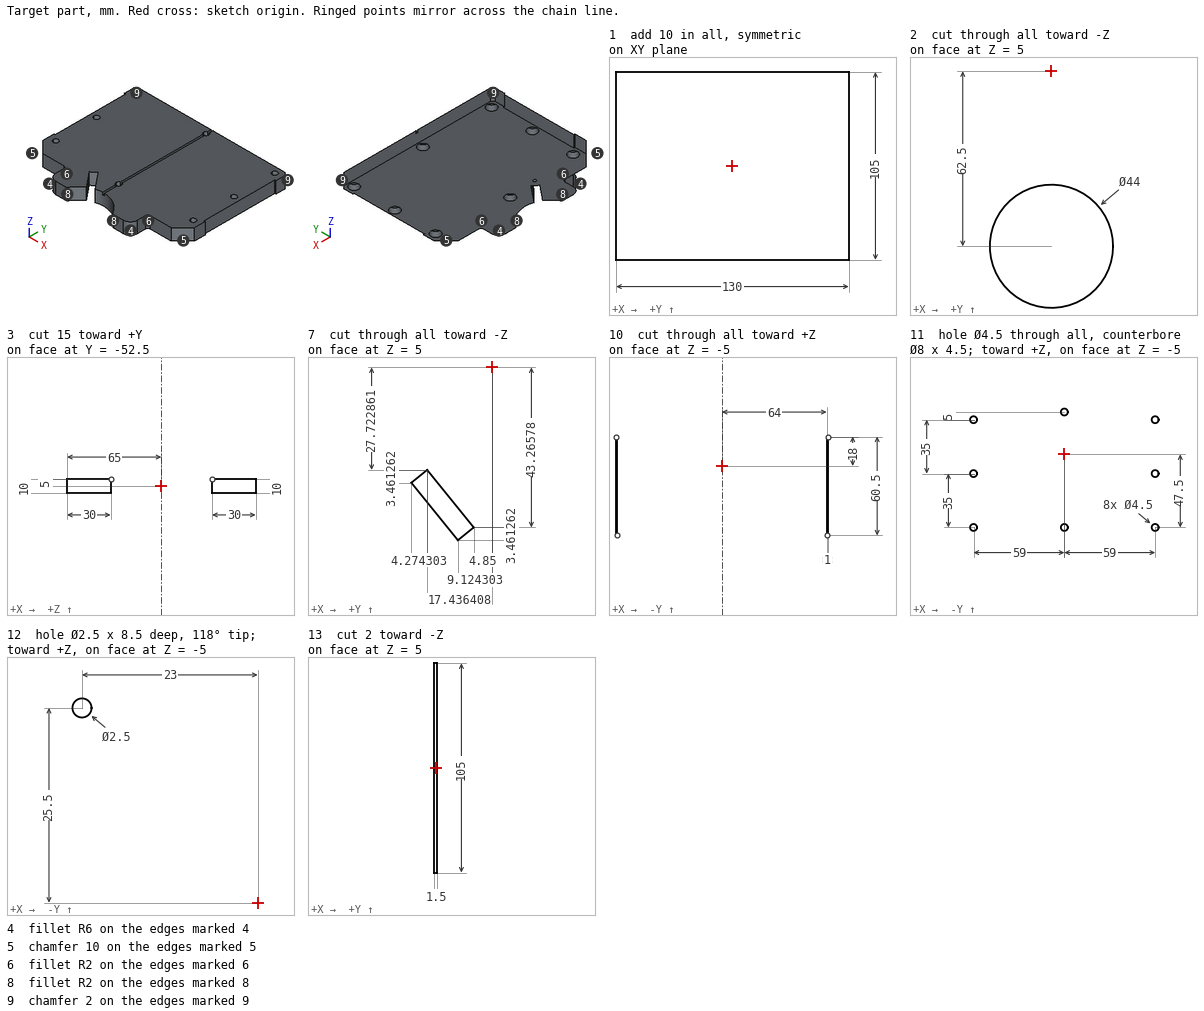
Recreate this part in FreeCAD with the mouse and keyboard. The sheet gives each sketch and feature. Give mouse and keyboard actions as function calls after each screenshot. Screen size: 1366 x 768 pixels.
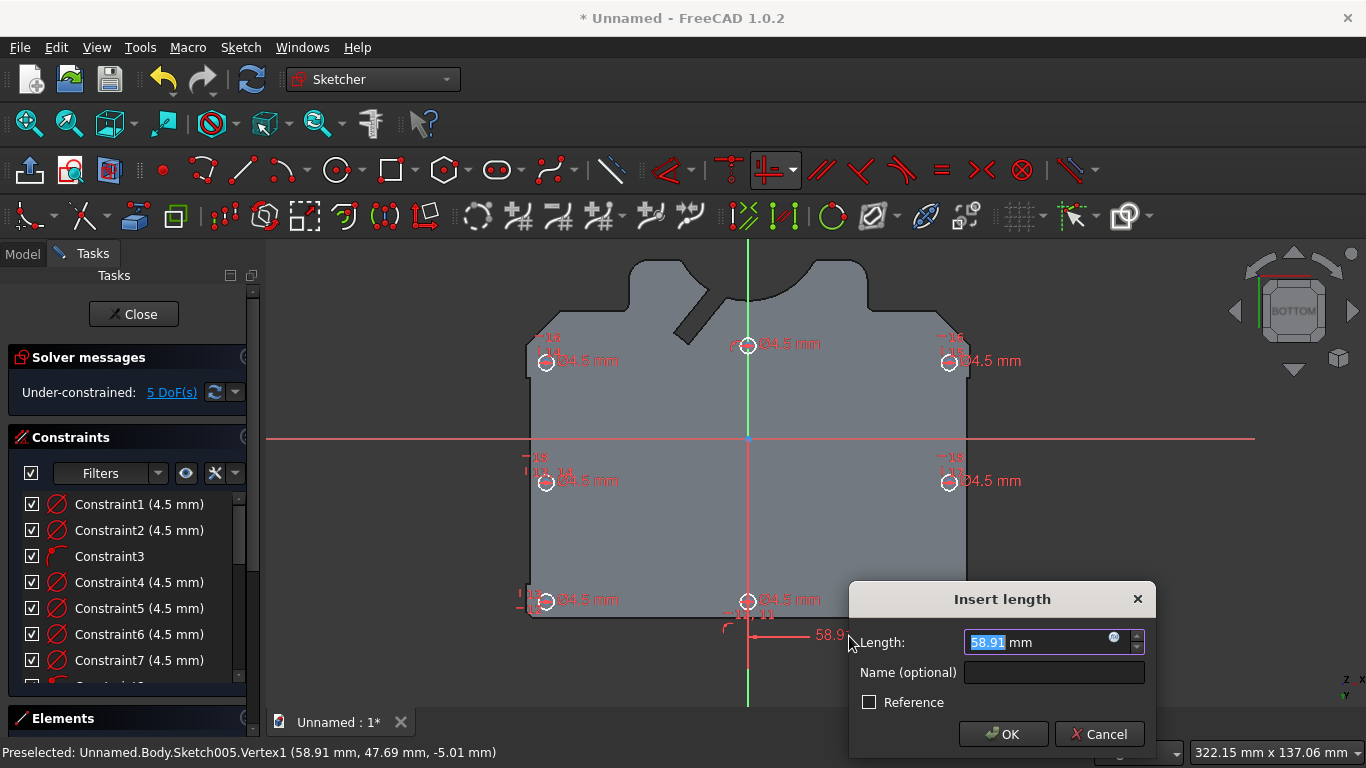
text(59)
key(Return)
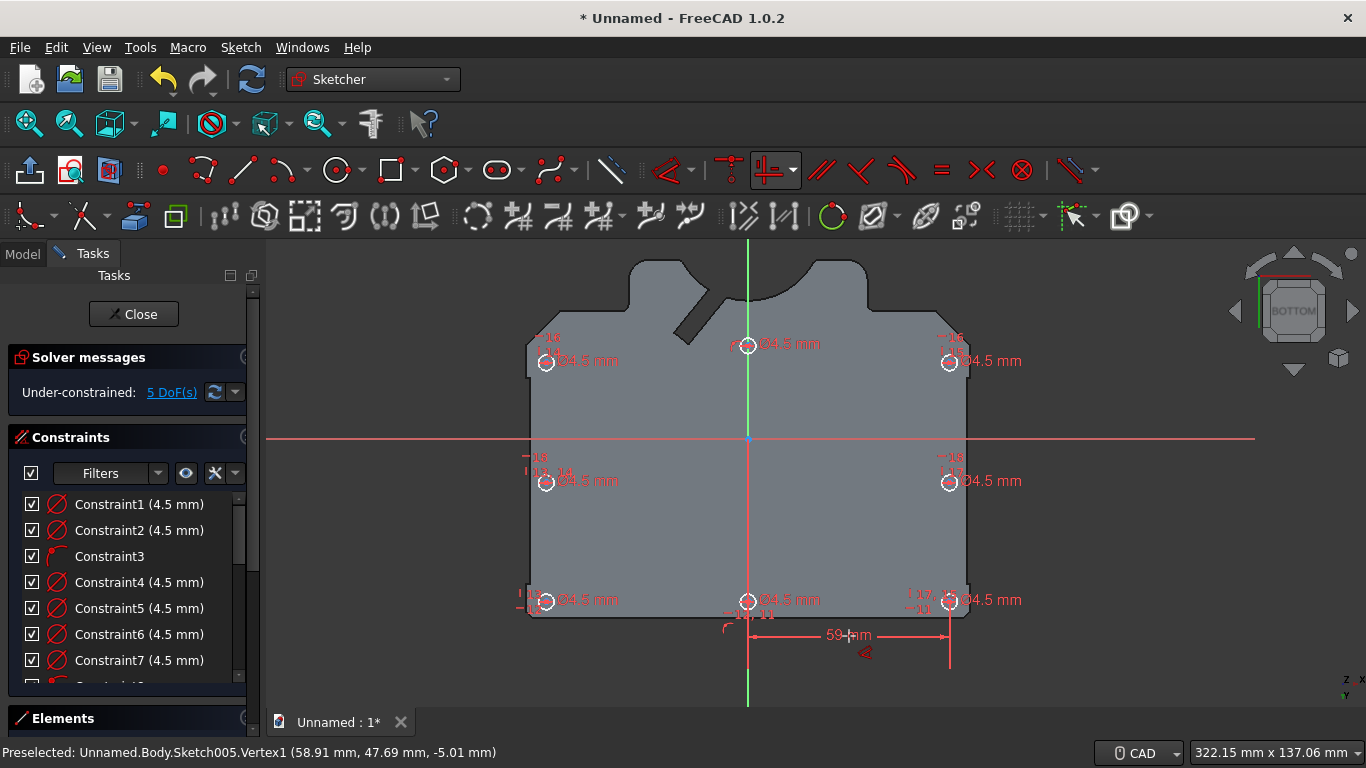
click(546, 602)
click(647, 636)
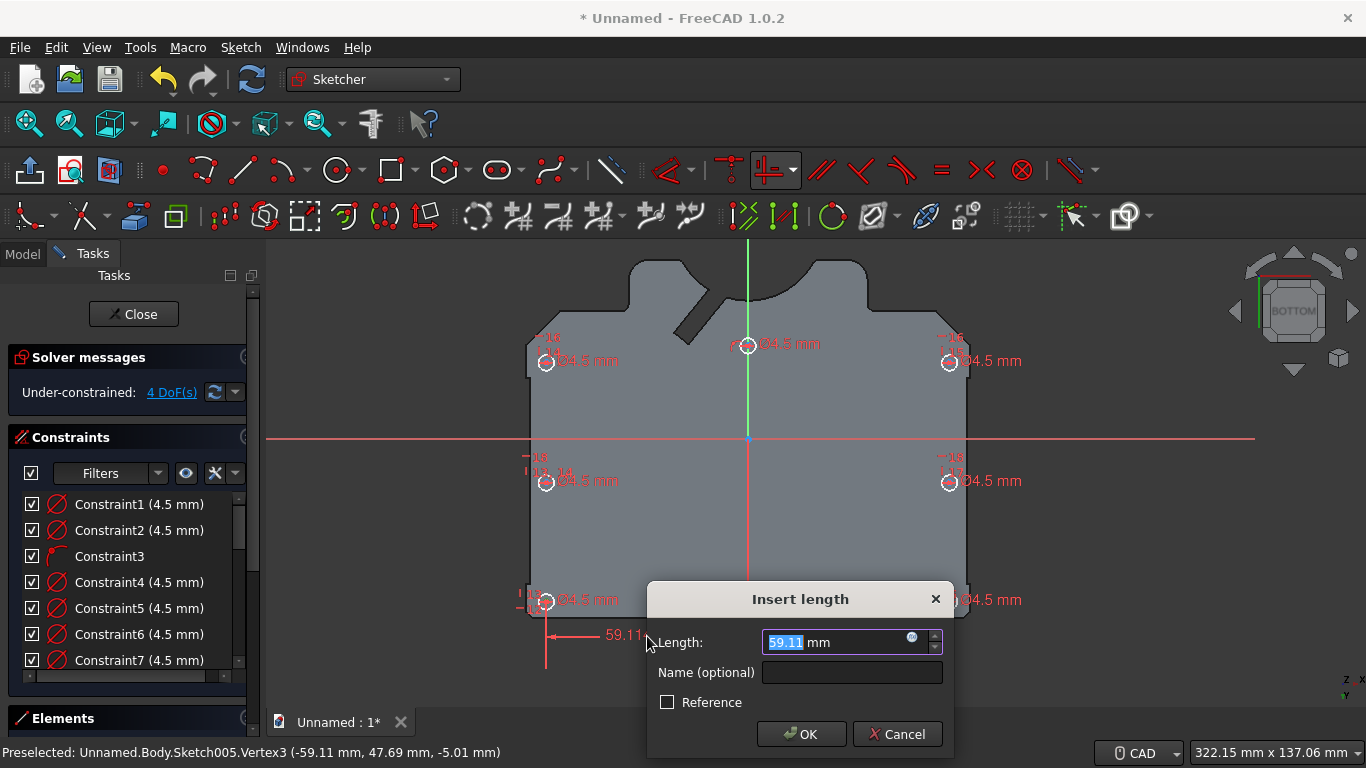
text(59)
key(Return)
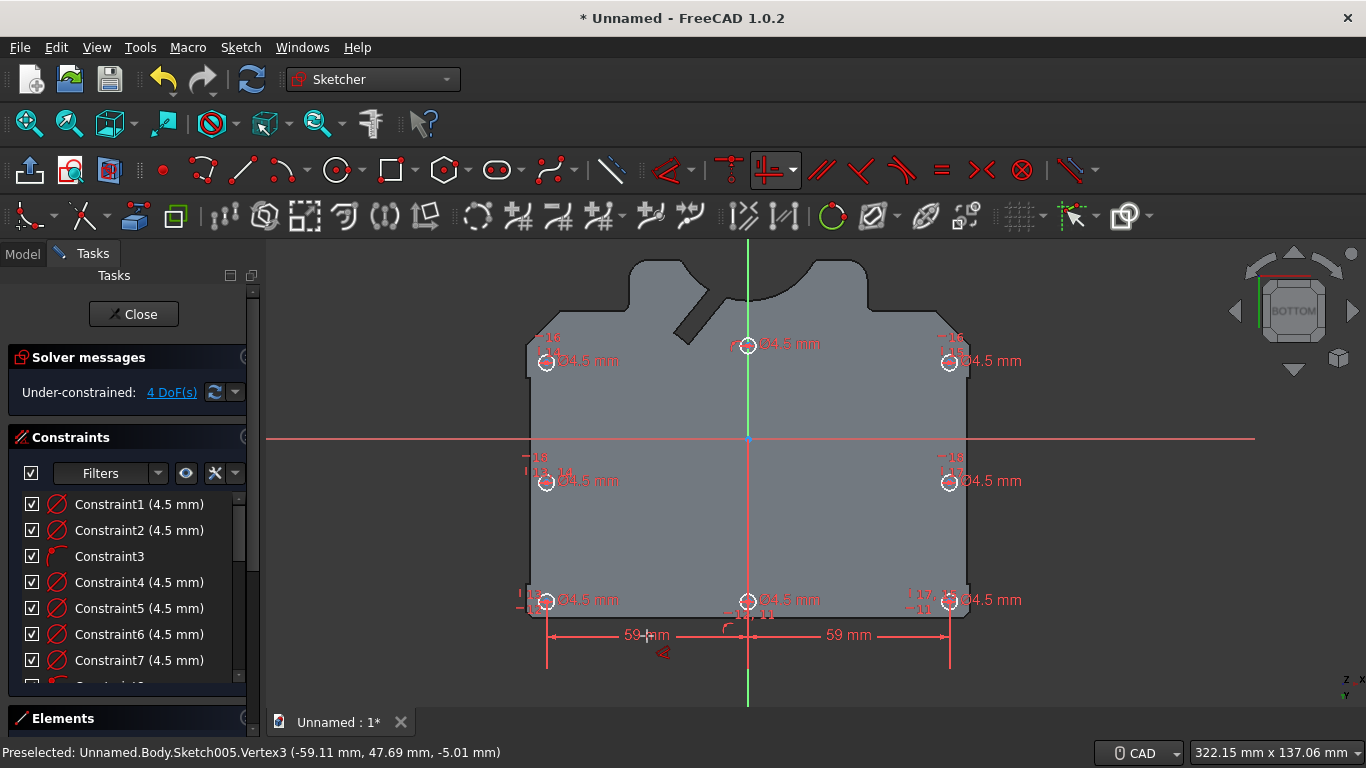
scroll(547, 363, up, 5)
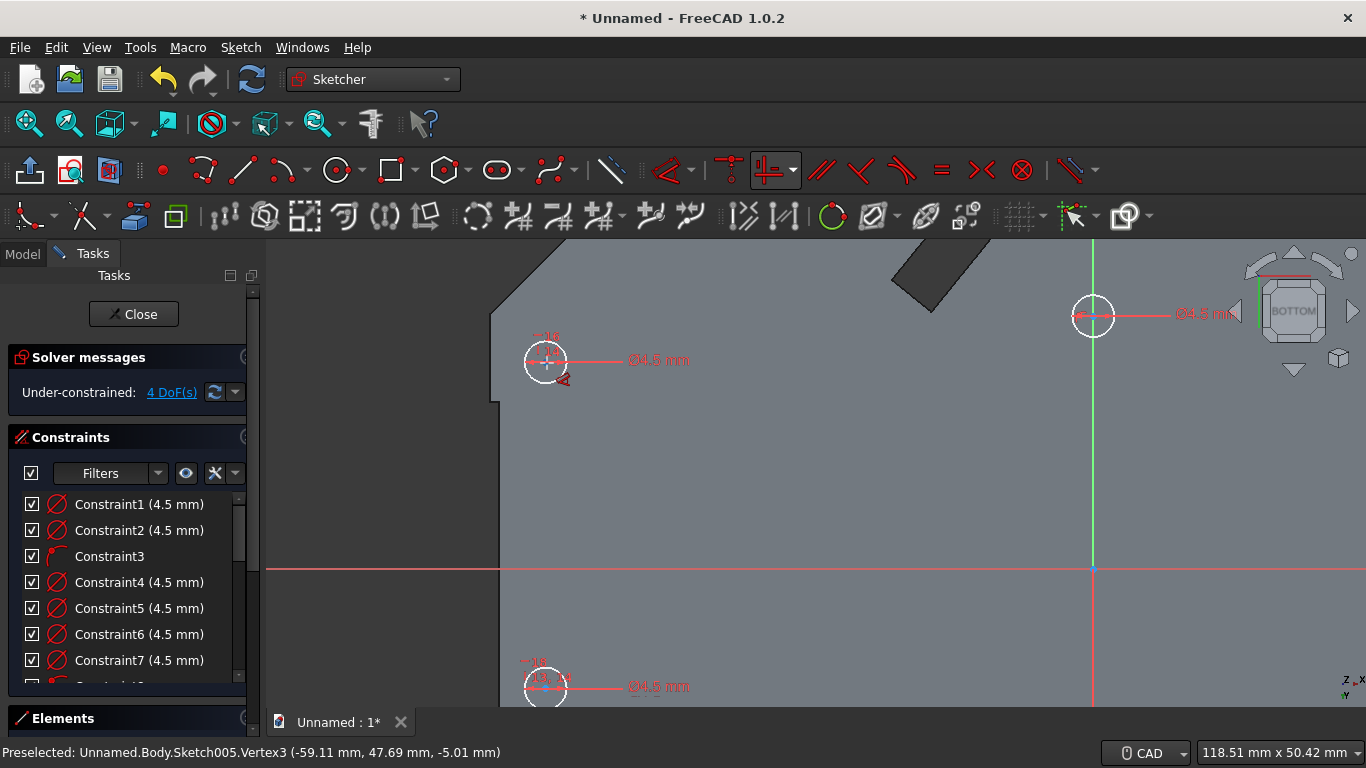
click(546, 362)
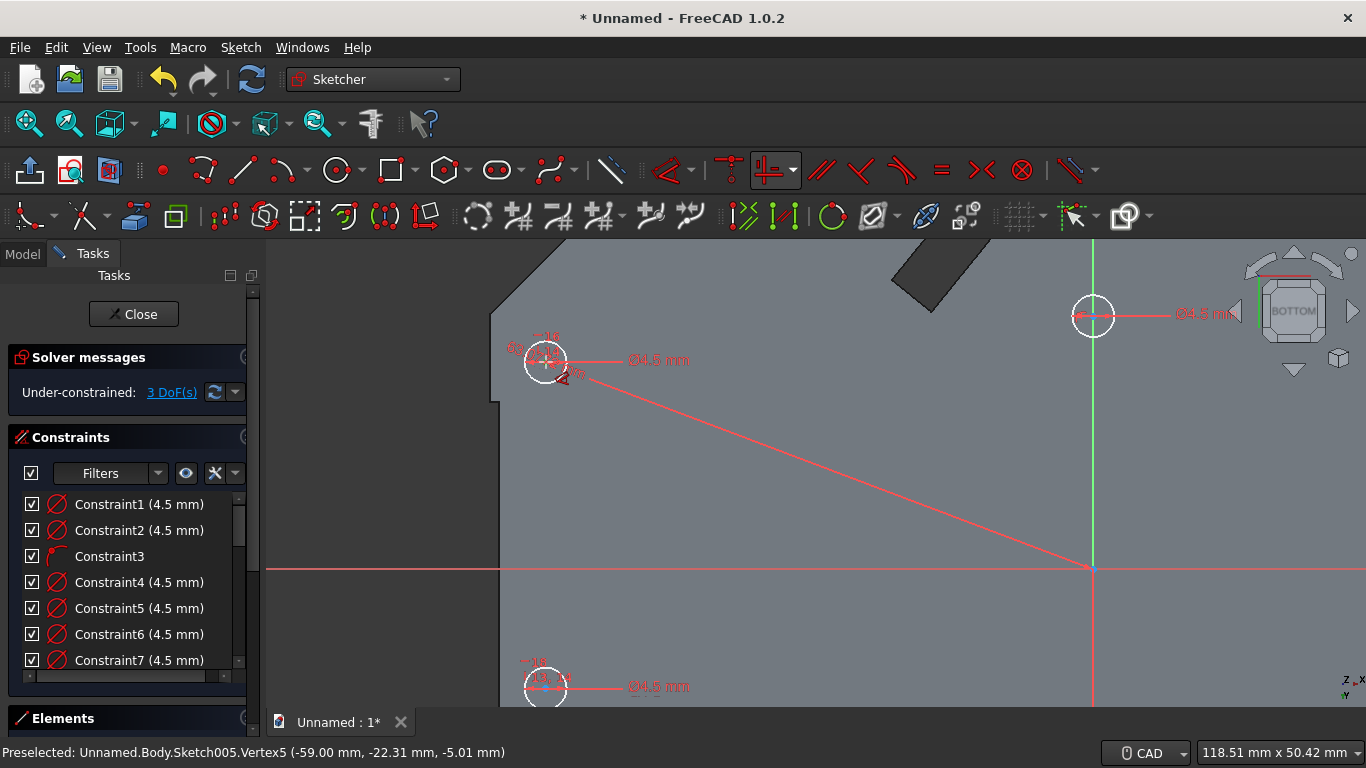
click(1093, 316)
click(512, 339)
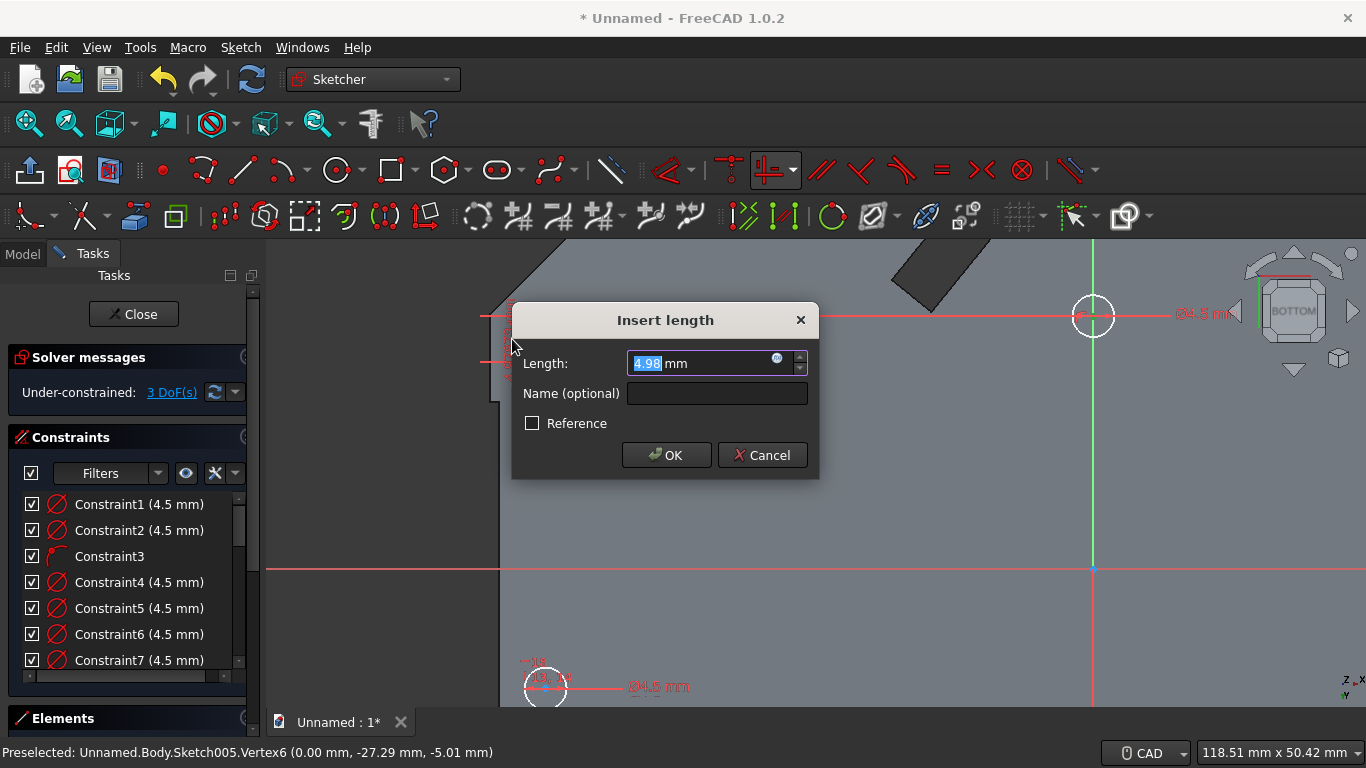
text(5)
key(Return)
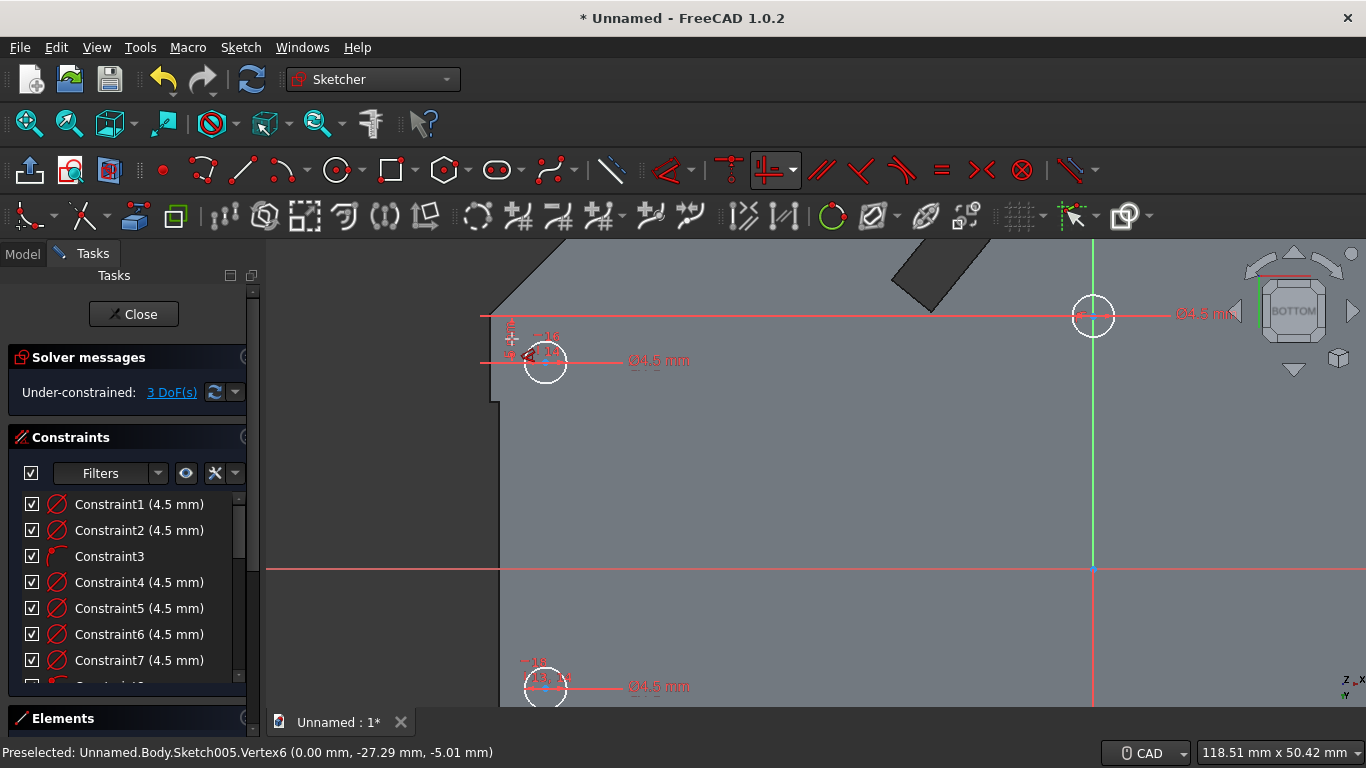
scroll(546, 363, down, 5)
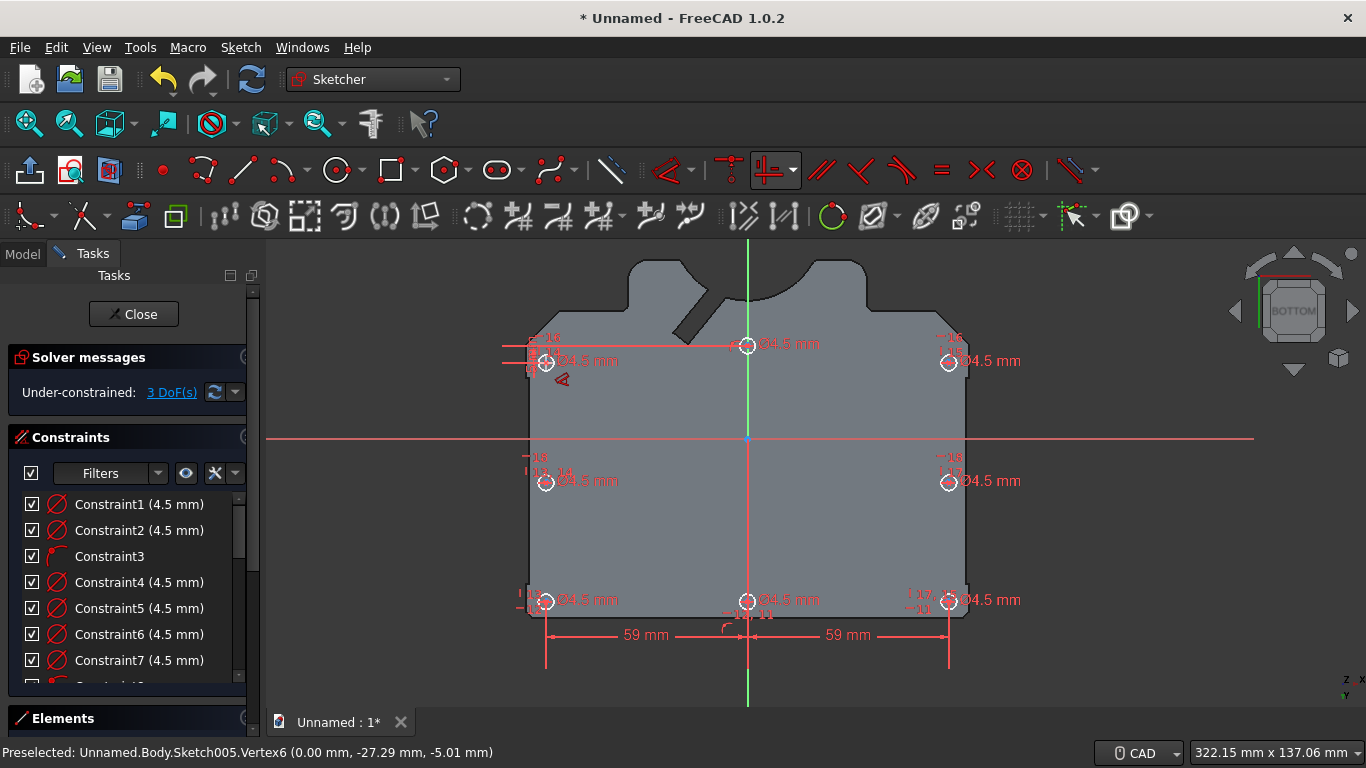
click(546, 602)